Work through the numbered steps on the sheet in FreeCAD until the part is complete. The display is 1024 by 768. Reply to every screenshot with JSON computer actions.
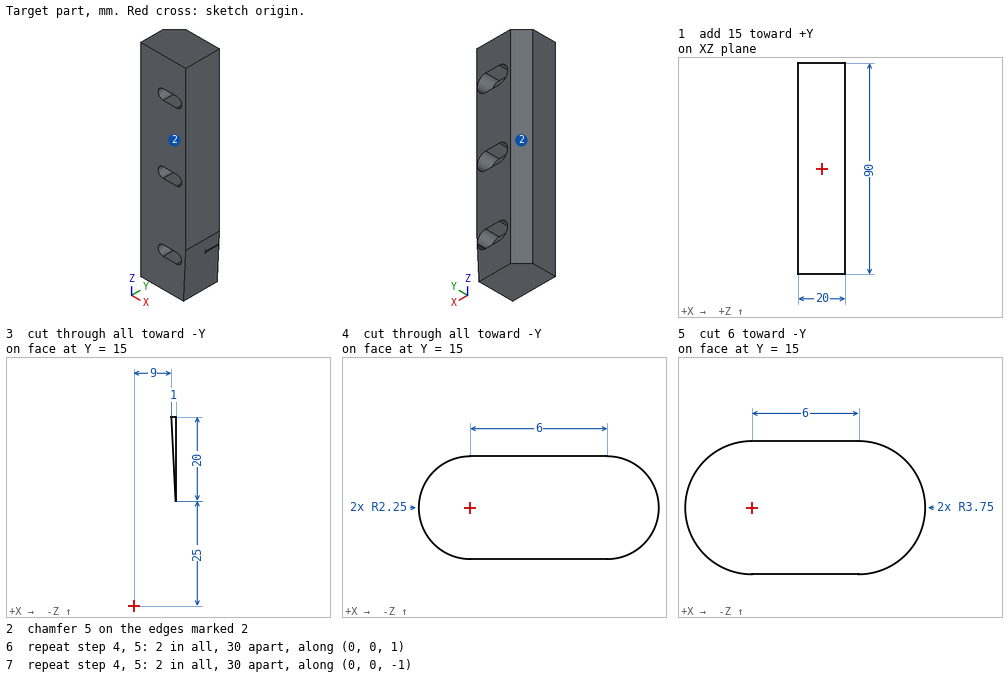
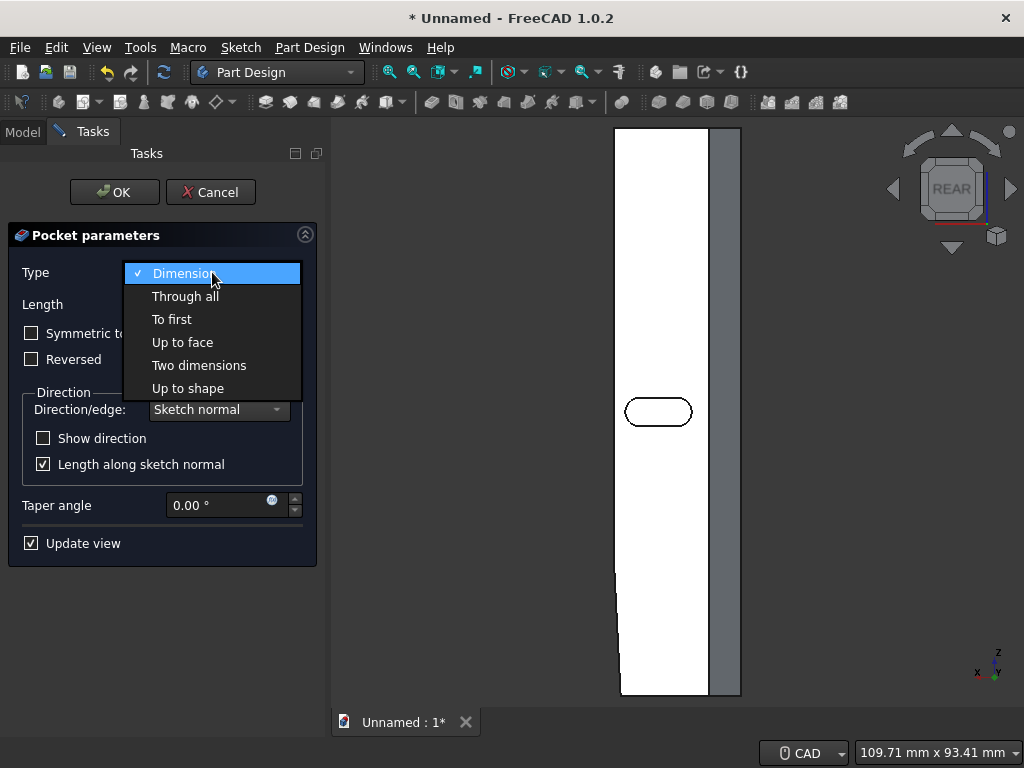
{"action": "left_click", "coordinate": [212, 296]}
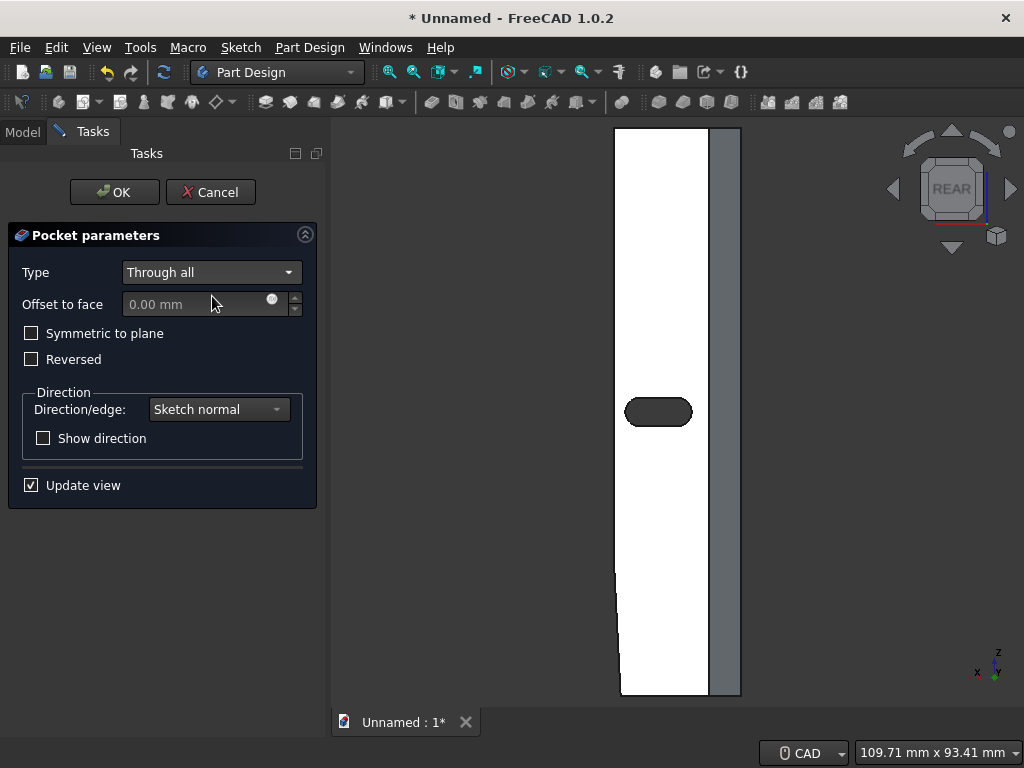
{"action": "left_click", "coordinate": [115, 192]}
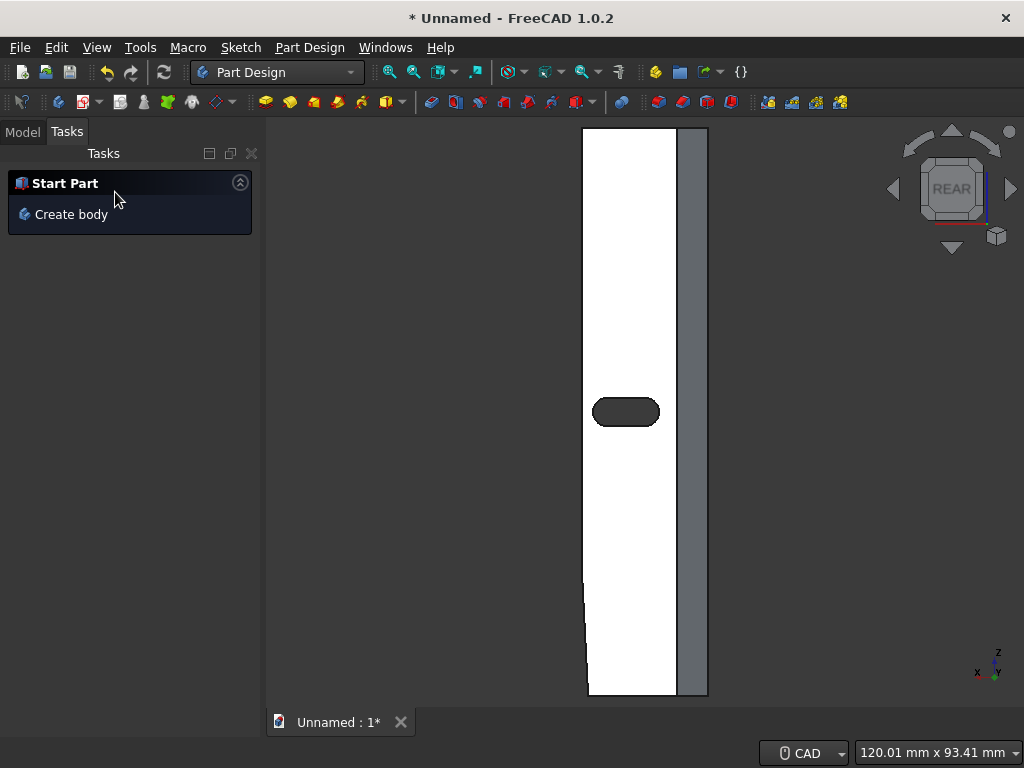
{"action": "left_click", "coordinate": [629, 249]}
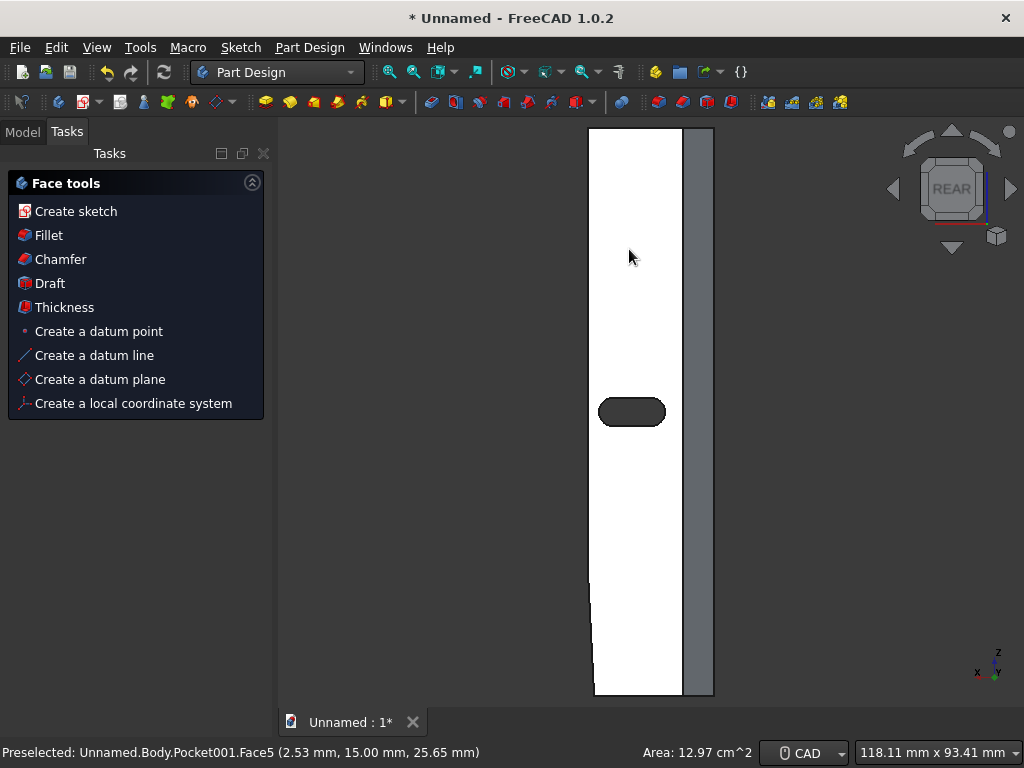
{"action": "left_click", "coordinate": [84, 102]}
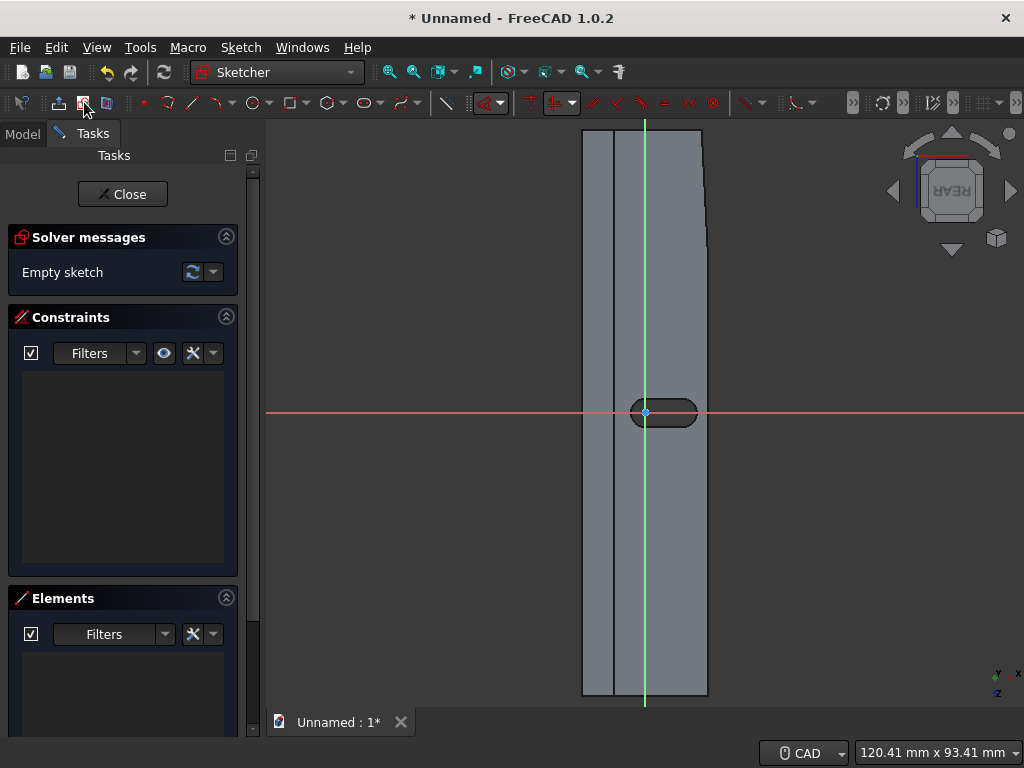
{"action": "scroll", "coordinate": [686, 413], "scroll_direction": "up", "scroll_amount": 8}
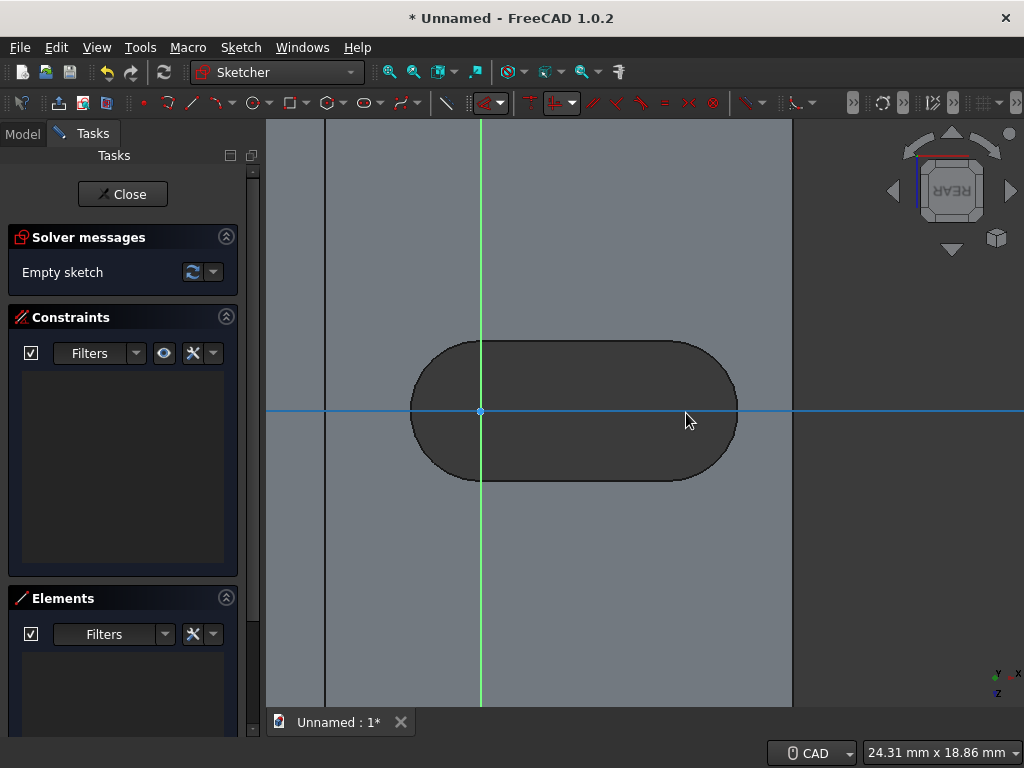
{"action": "left_click", "coordinate": [364, 104]}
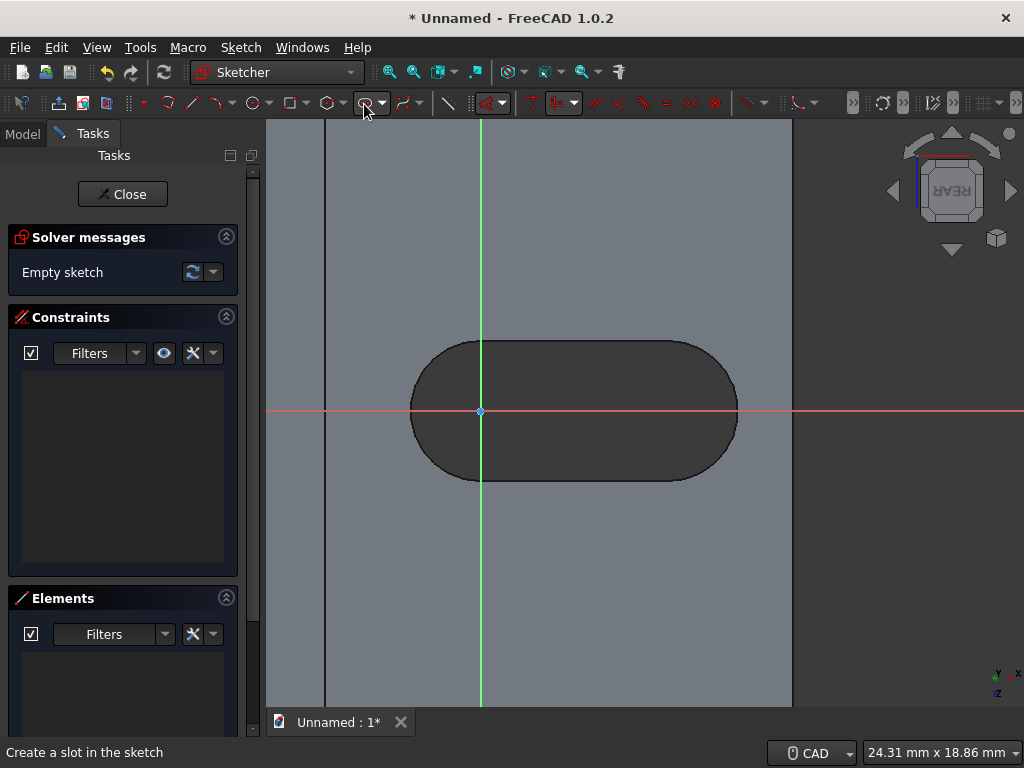
{"action": "left_click", "coordinate": [481, 411]}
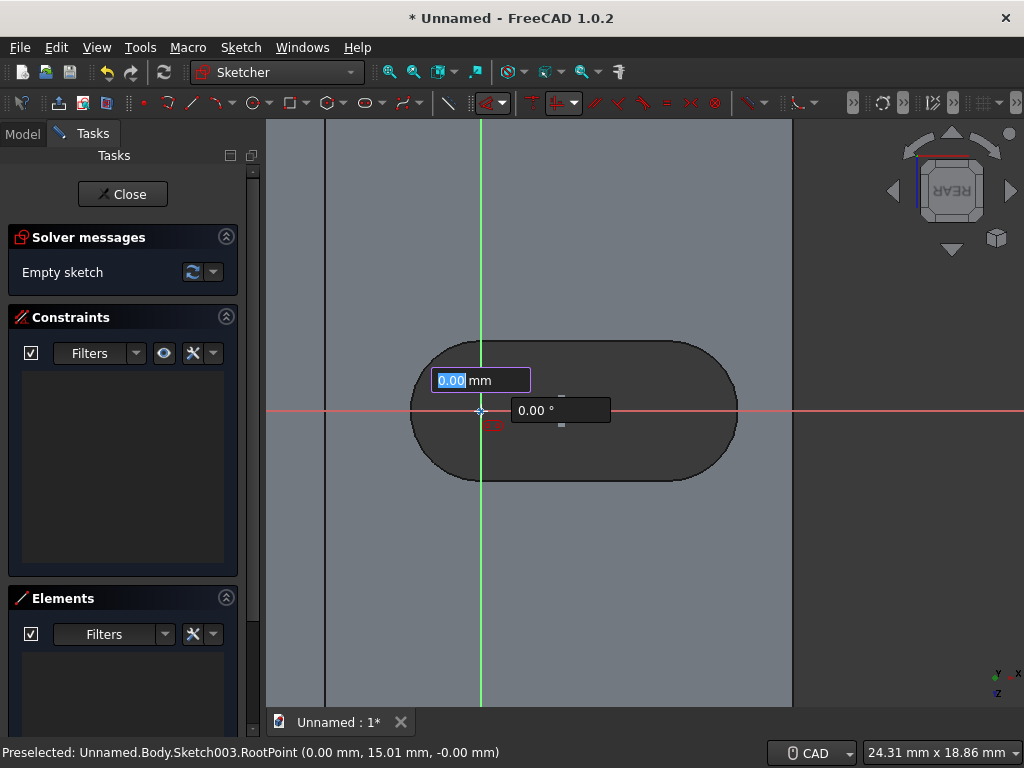
{"action": "left_click", "coordinate": [668, 402]}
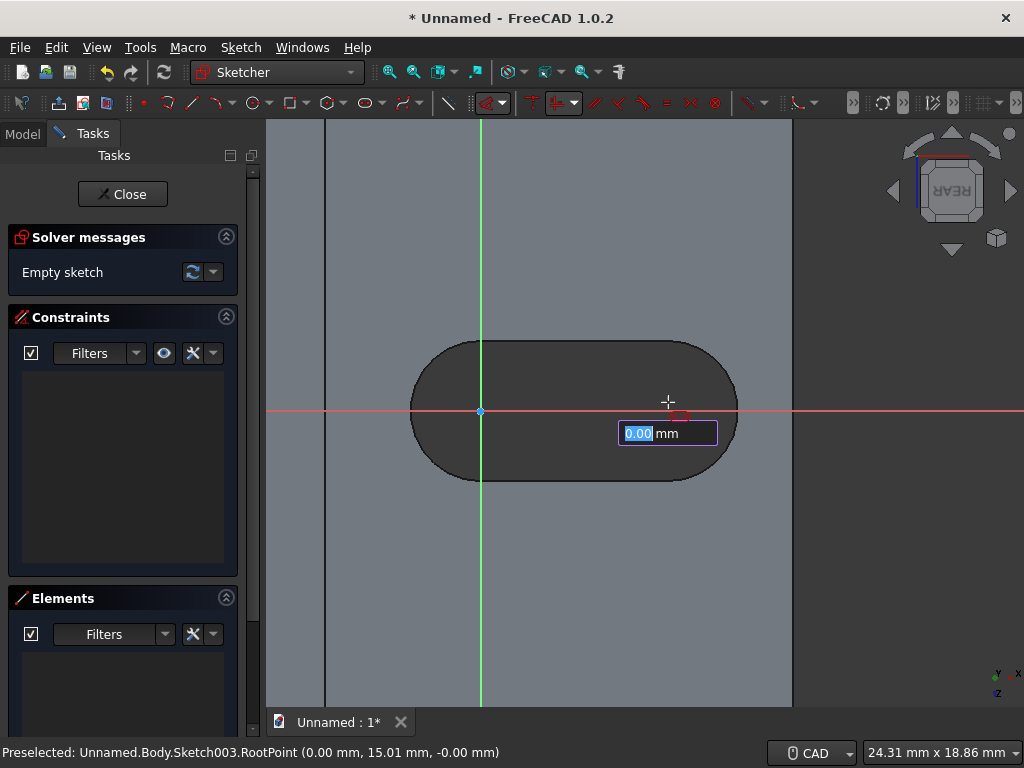
{"action": "left_click", "coordinate": [574, 528]}
{"action": "key", "text": "Escape"}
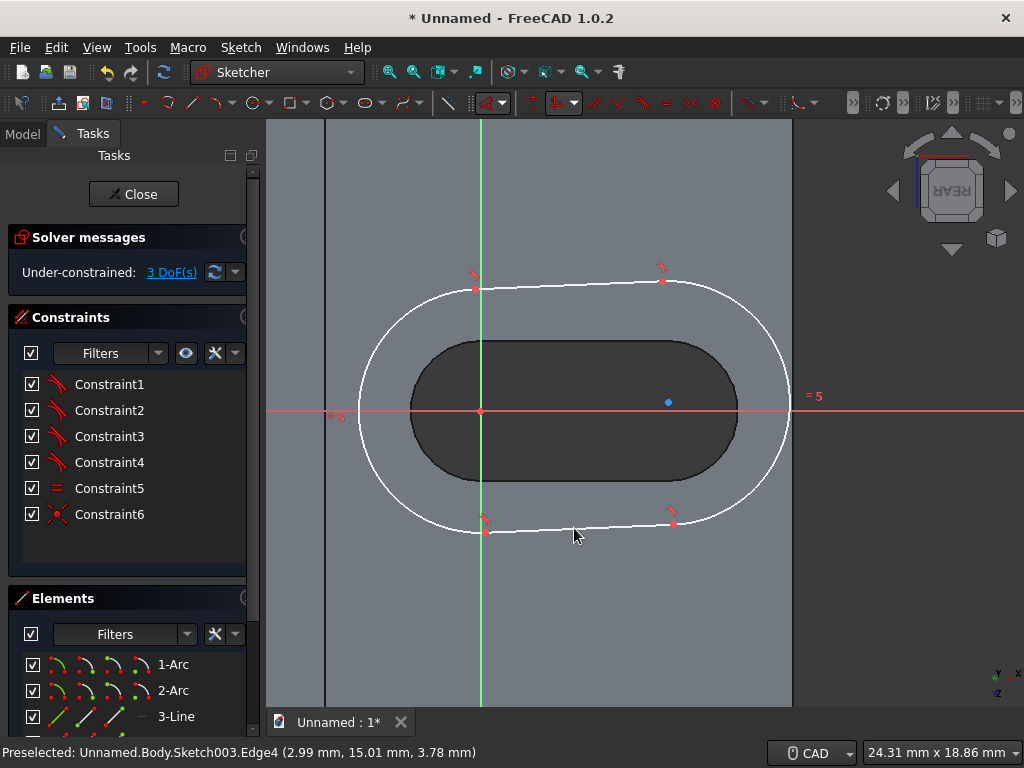
{"action": "left_click", "coordinate": [532, 287]}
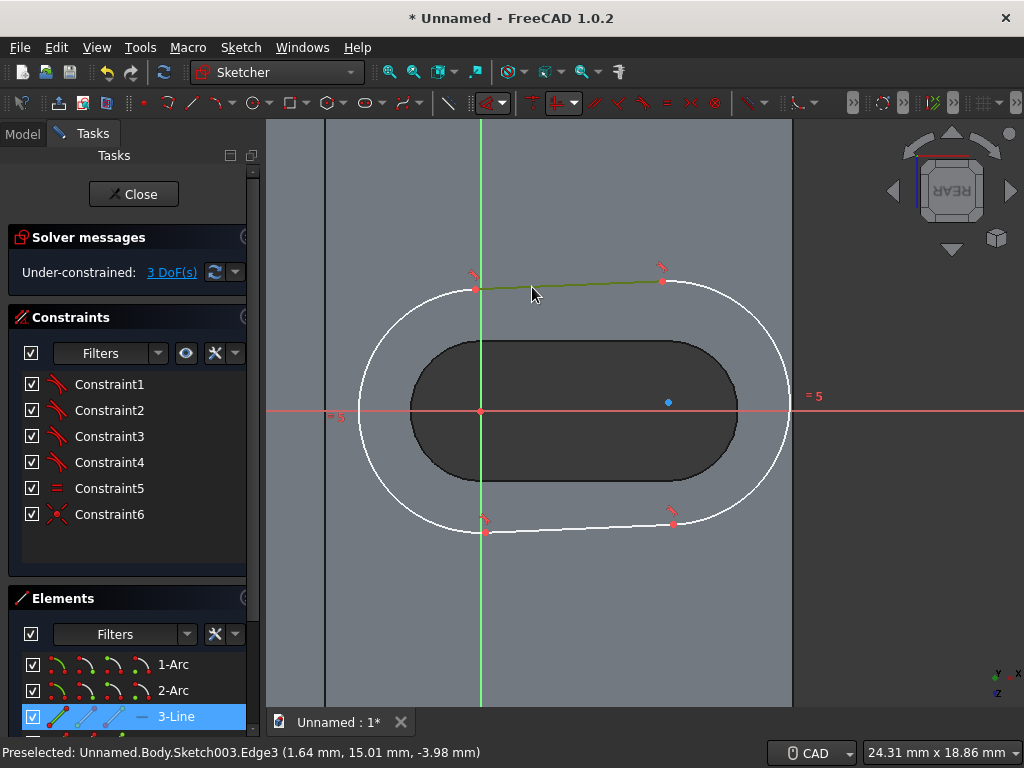
{"action": "left_click", "coordinate": [576, 104]}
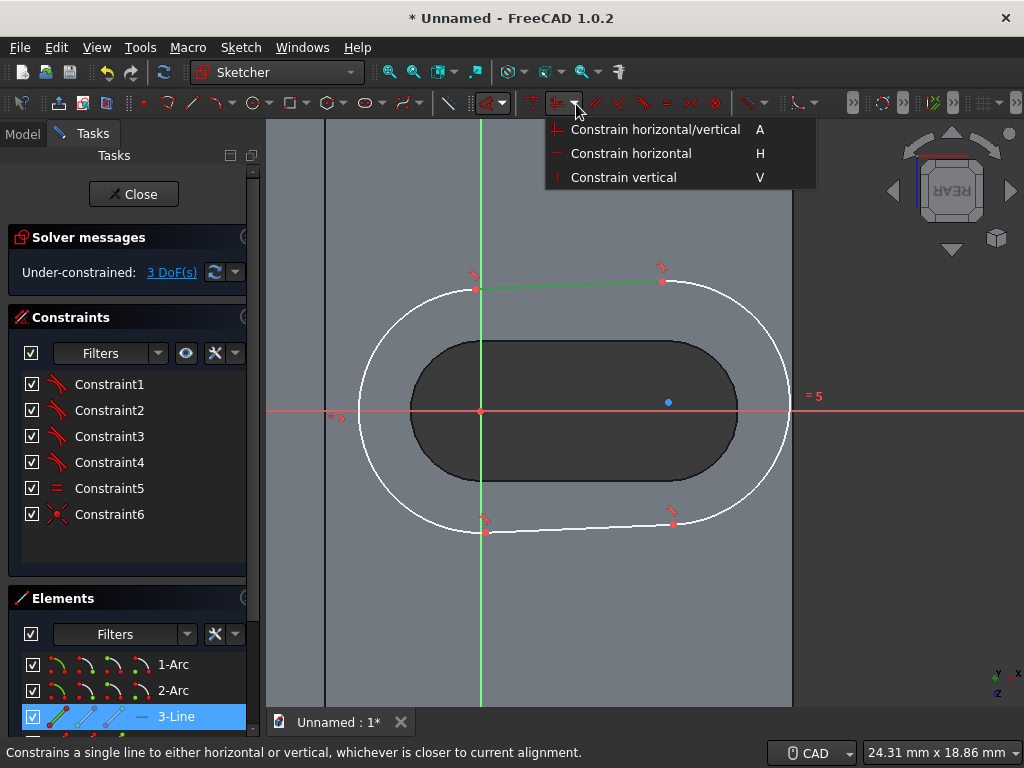
{"action": "left_click", "coordinate": [681, 153]}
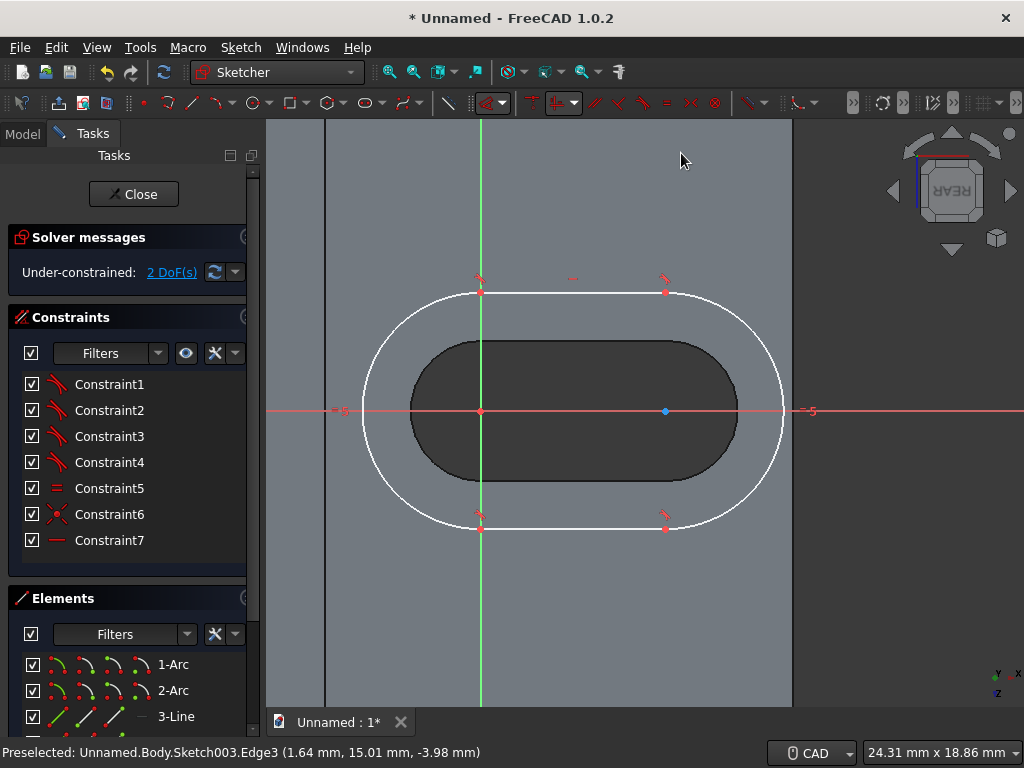
{"action": "left_click", "coordinate": [385, 342]}